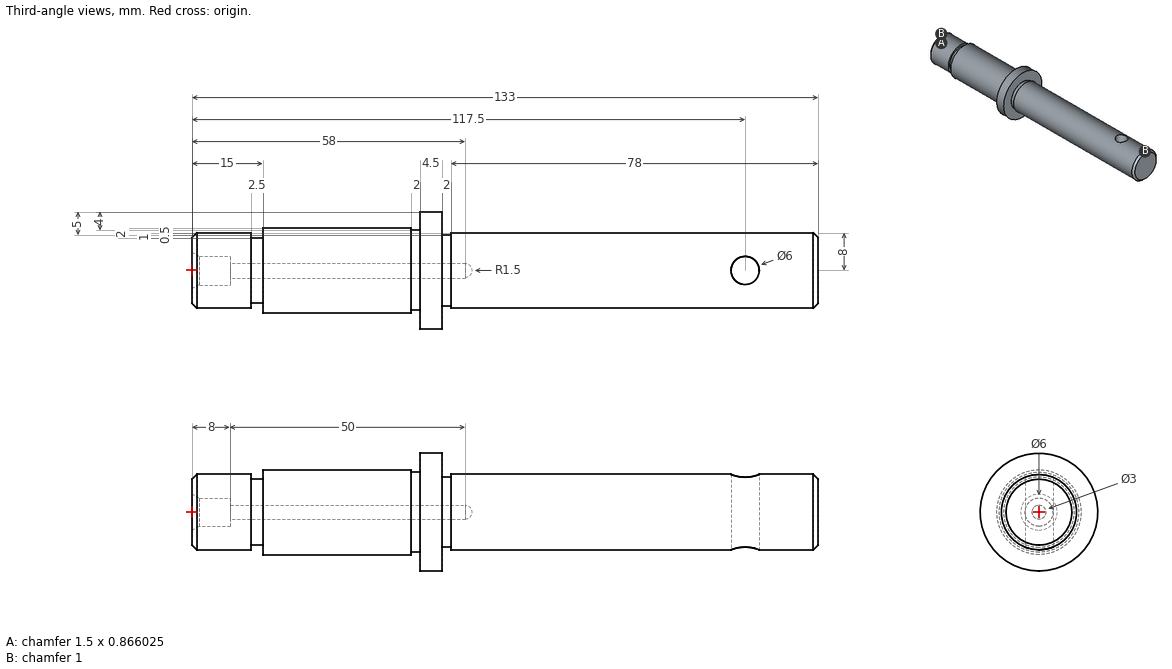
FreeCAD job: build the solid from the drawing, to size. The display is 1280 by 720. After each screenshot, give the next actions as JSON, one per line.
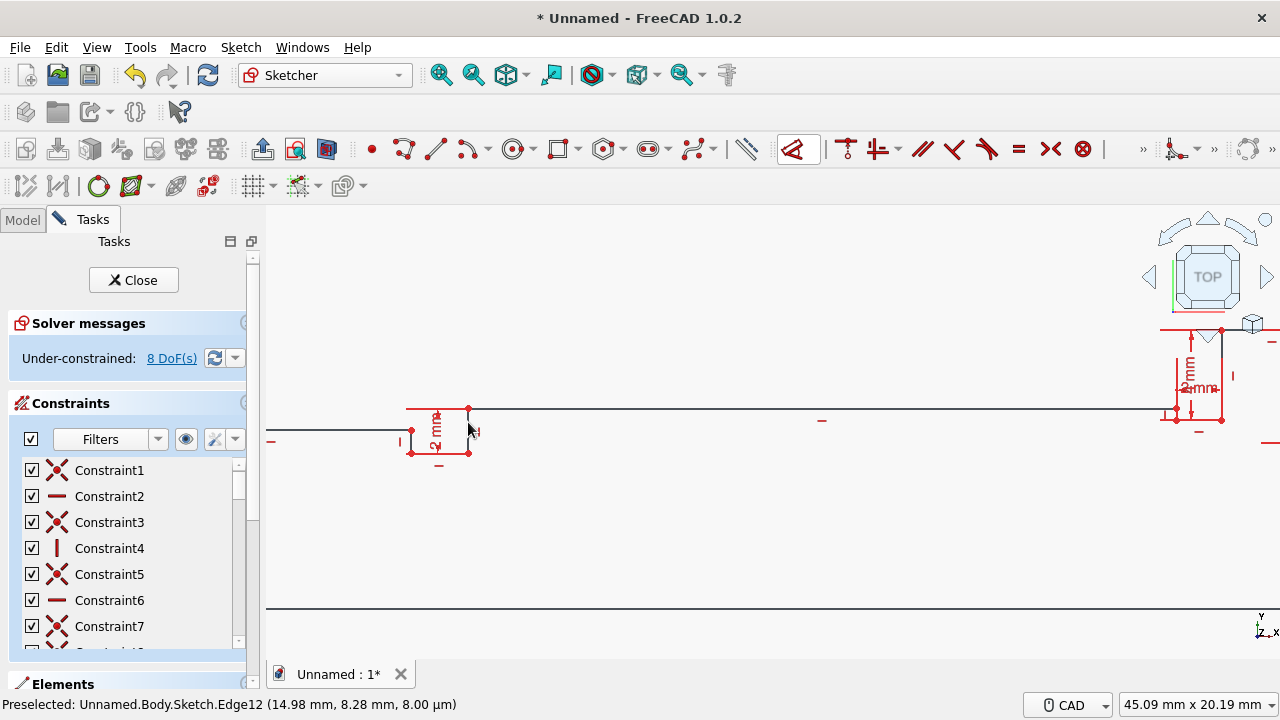
{"action": "scroll", "coordinate": [411, 444], "scroll_direction": "up", "scroll_amount": 3}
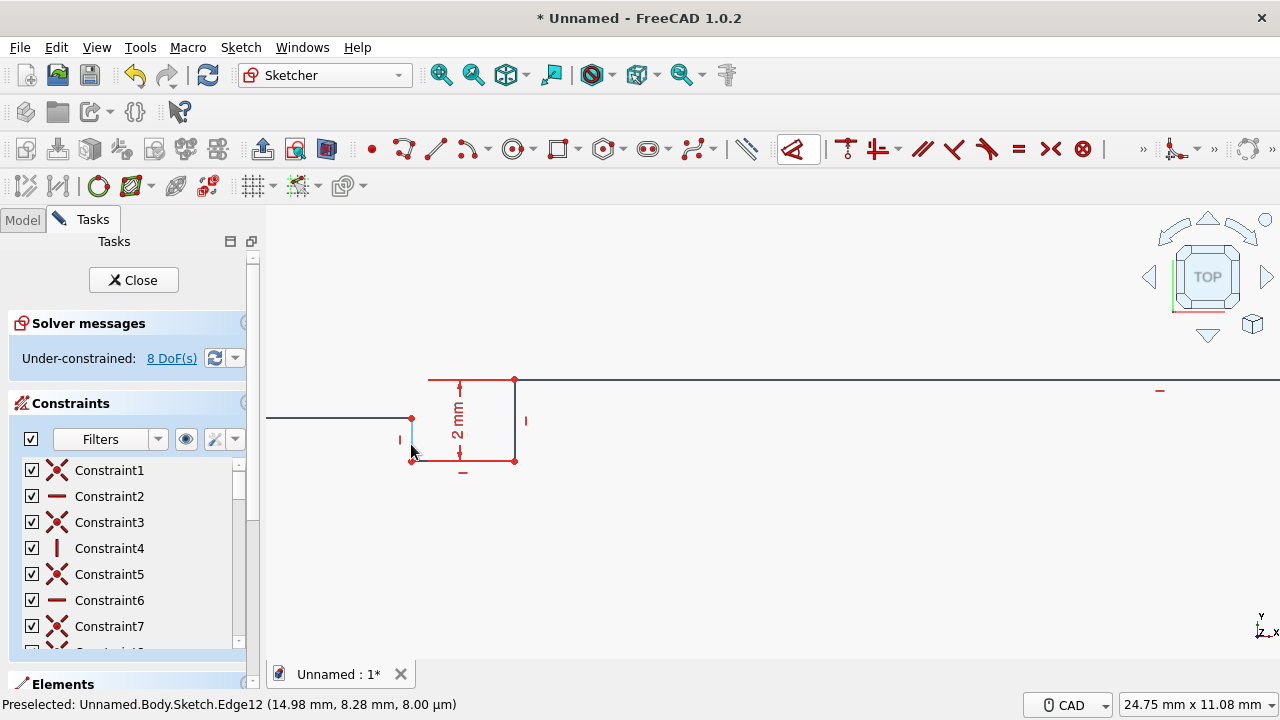
{"action": "left_click", "coordinate": [412, 444]}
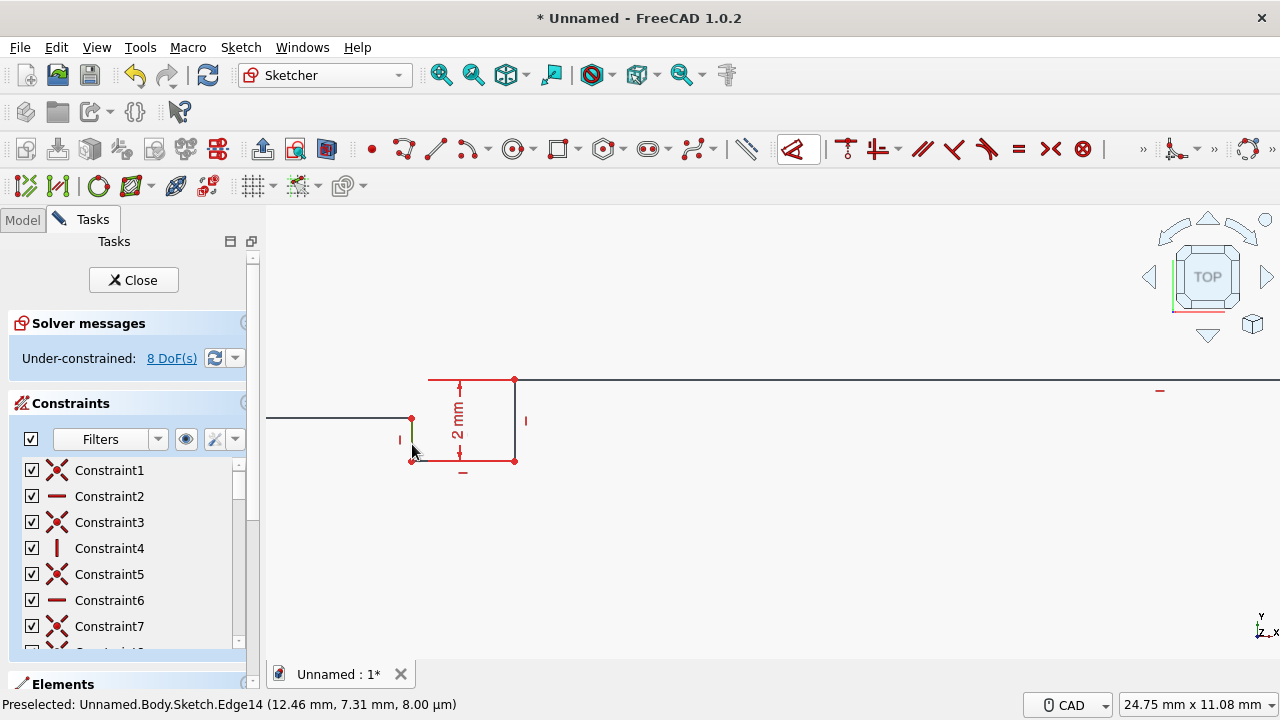
{"action": "key", "text": "i"}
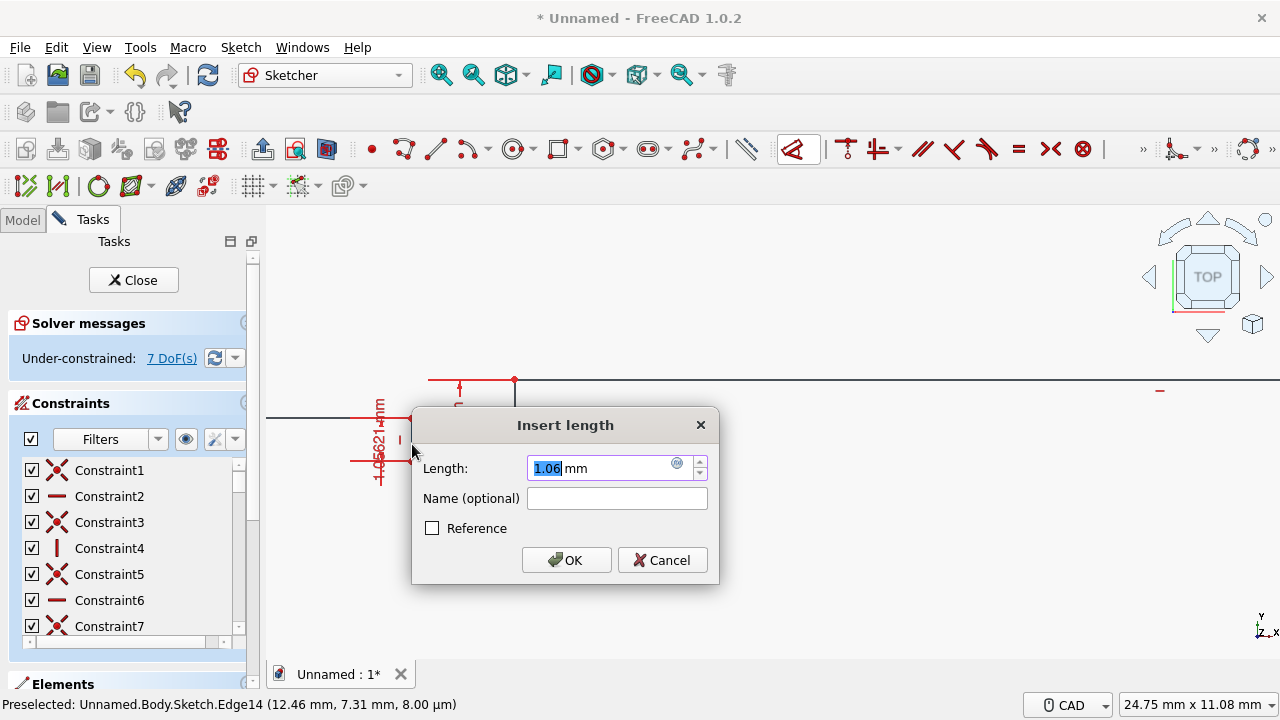
{"action": "type", "text": "1"}
{"action": "key", "text": "Return"}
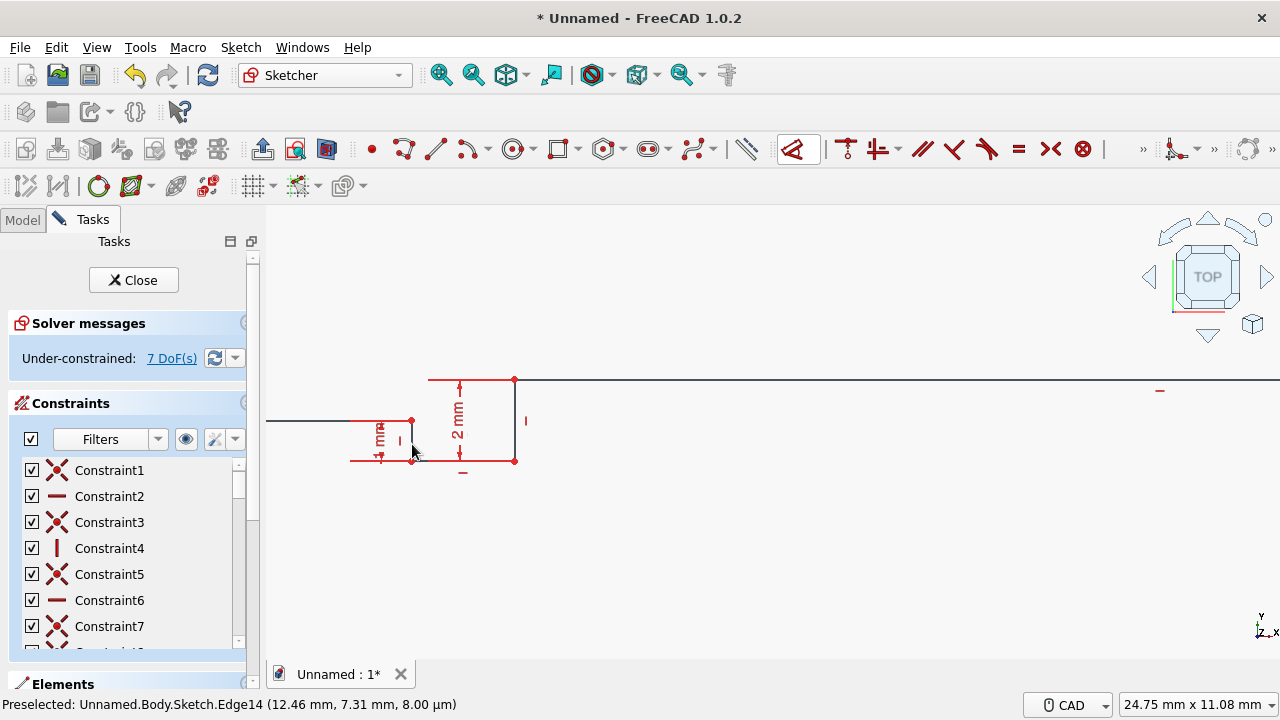
{"action": "scroll", "coordinate": [465, 425], "scroll_direction": "down", "scroll_amount": 11}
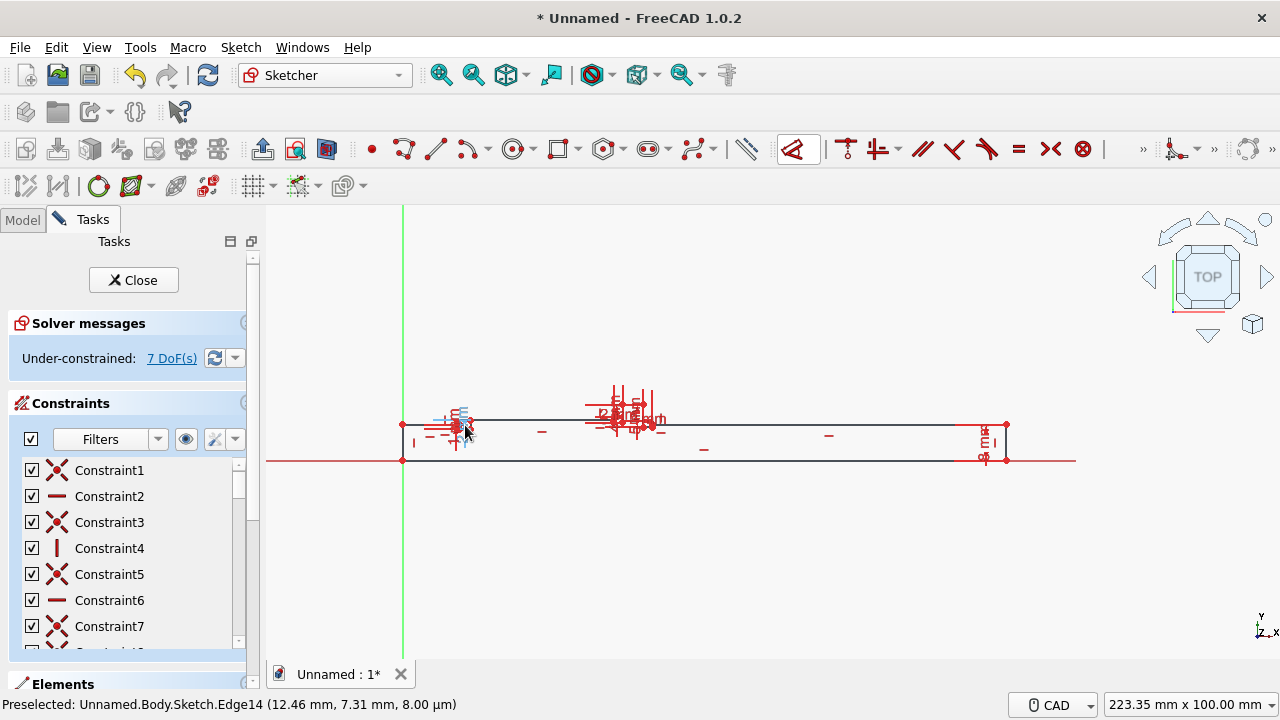
{"action": "scroll", "coordinate": [403, 436], "scroll_direction": "up", "scroll_amount": 2}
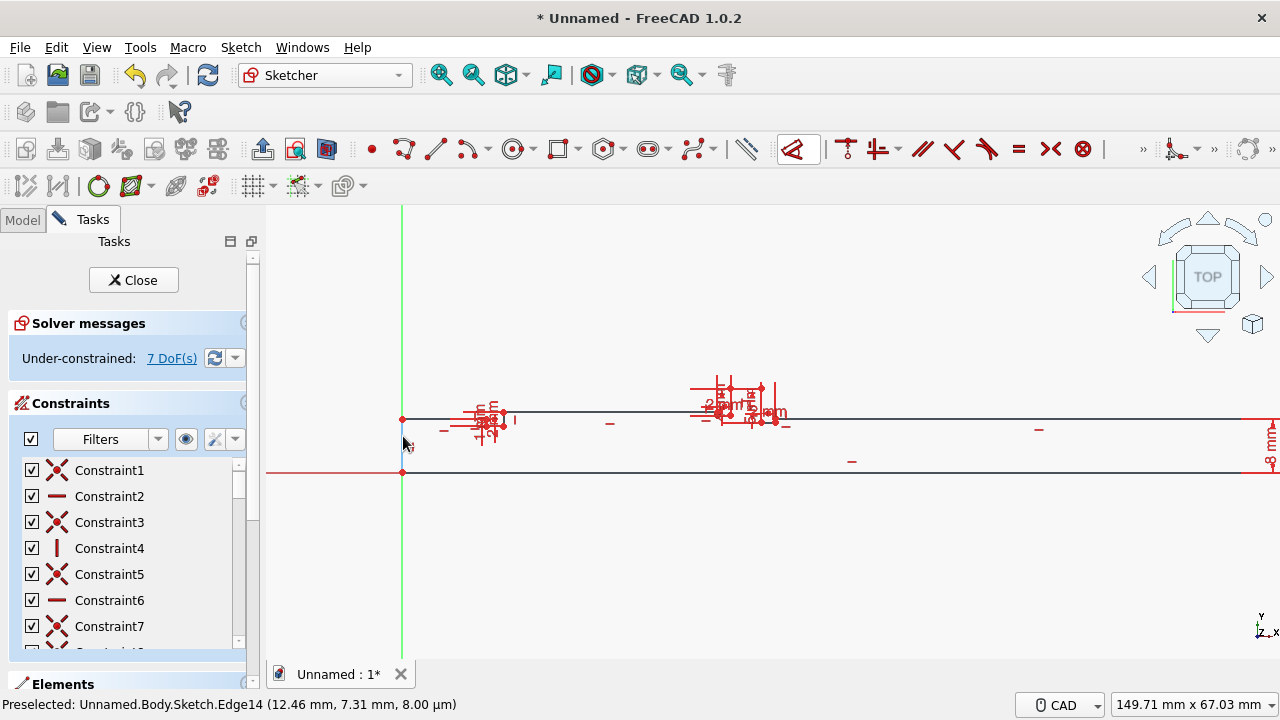
{"action": "left_click", "coordinate": [402, 435]}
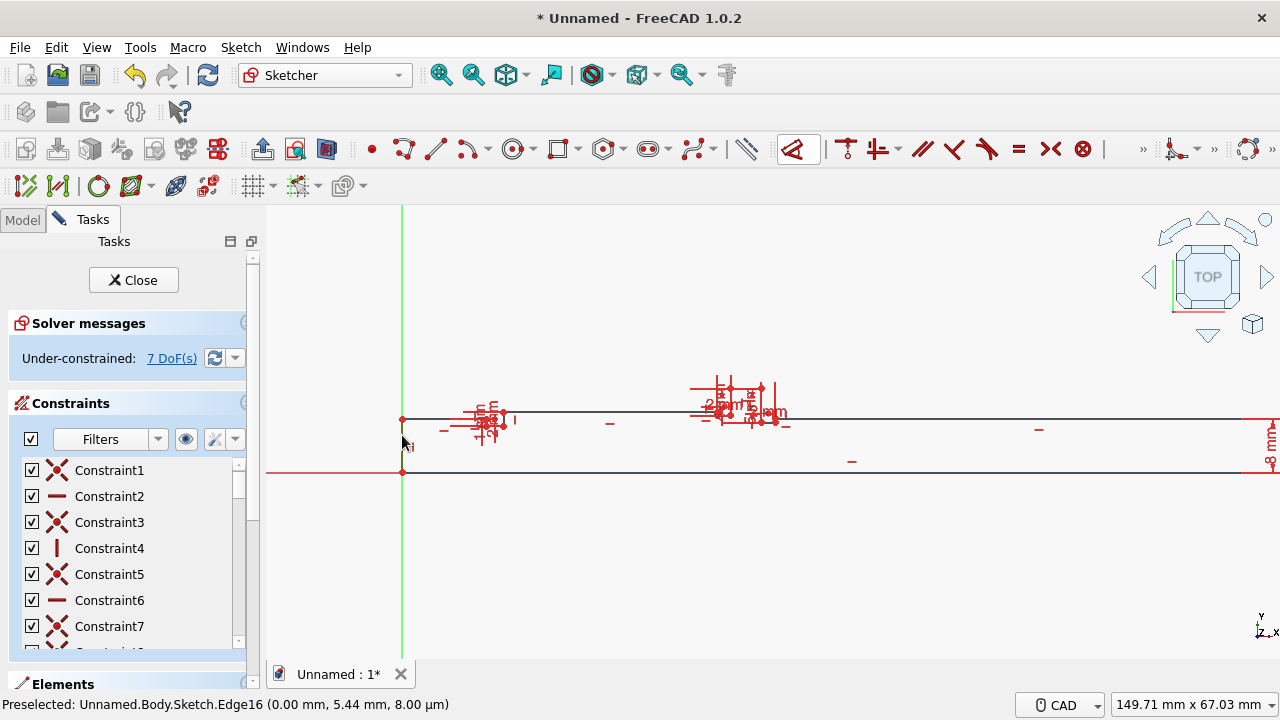
{"action": "left_click", "coordinate": [814, 150]}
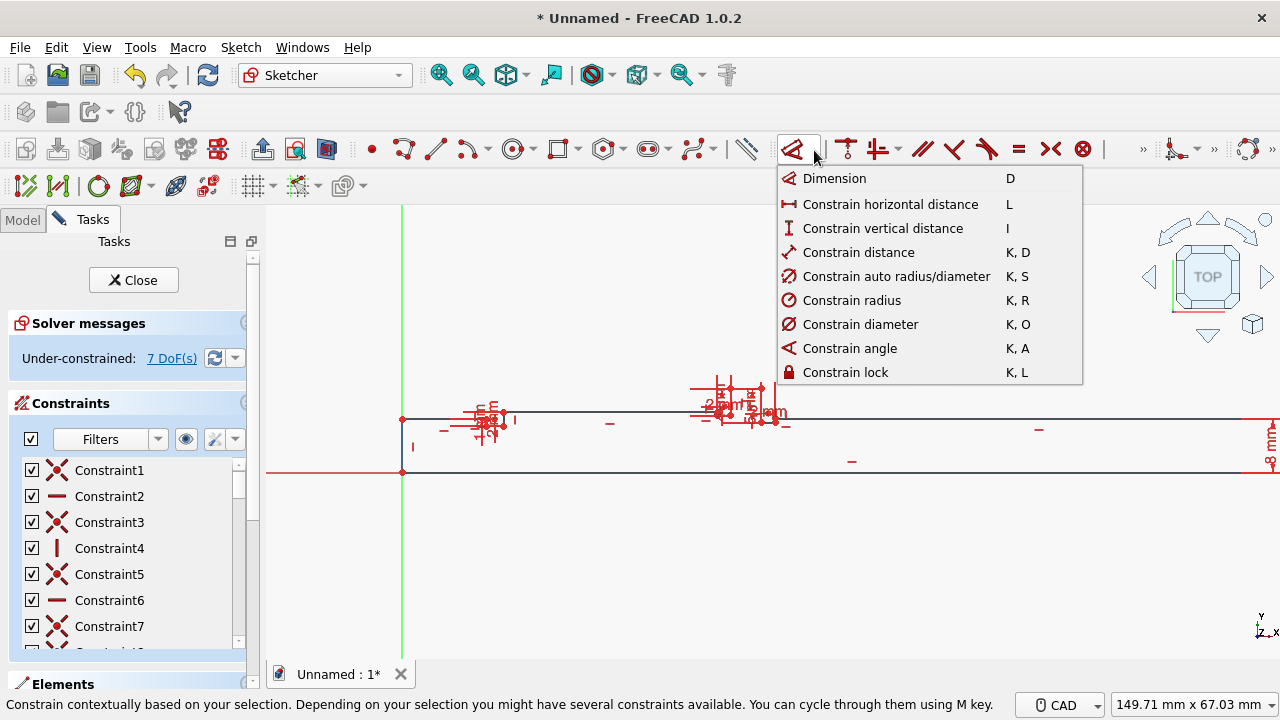
{"action": "left_click", "coordinate": [930, 228]}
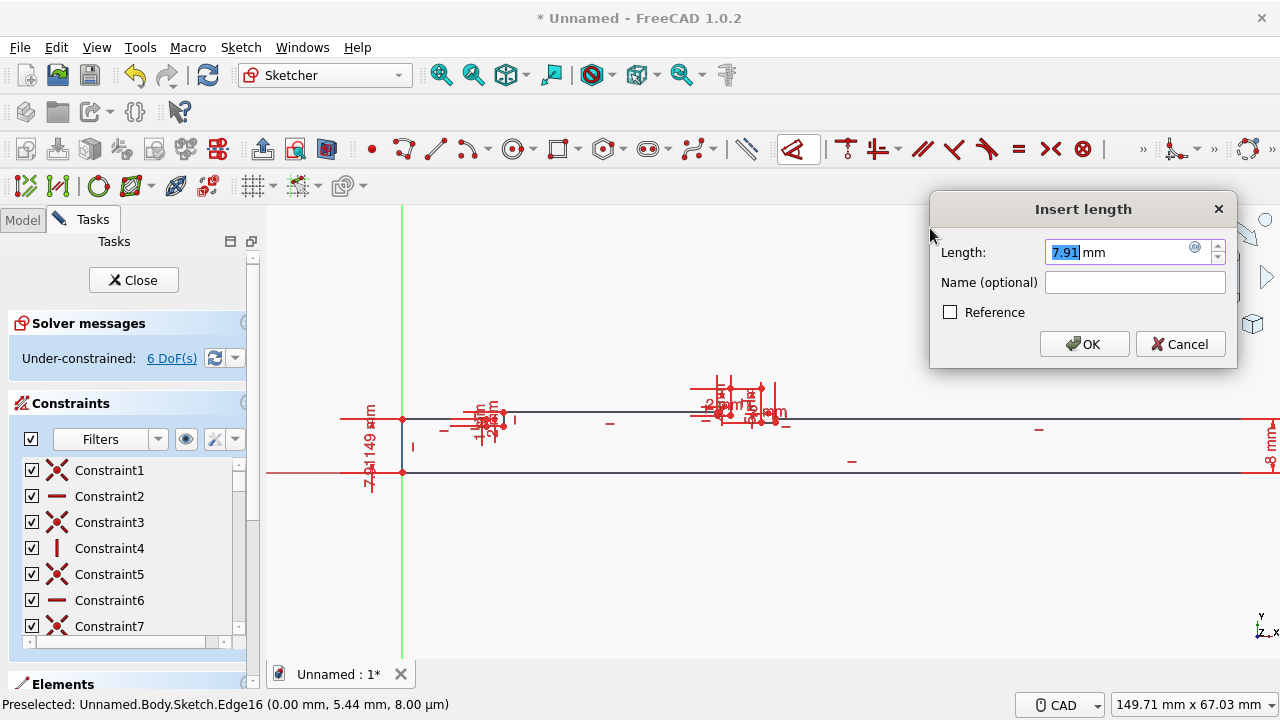
{"action": "type", "text": "8"}
{"action": "key", "text": "Return"}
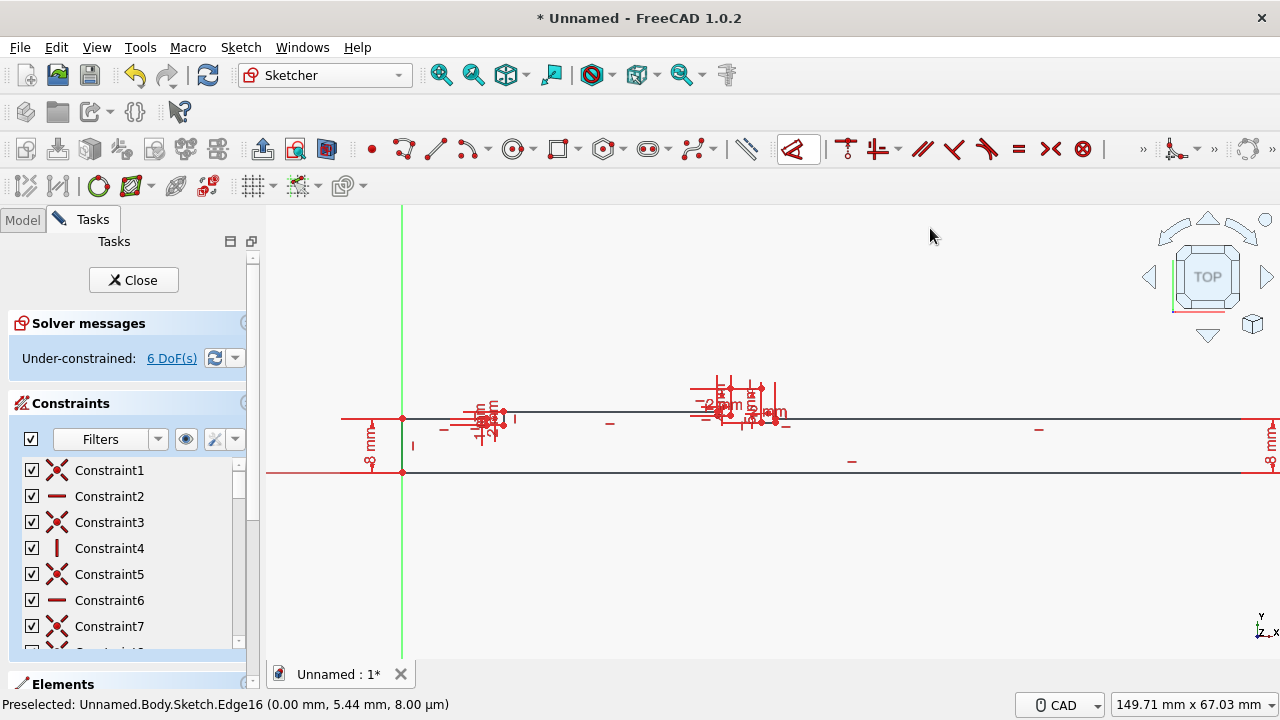
{"action": "left_click", "coordinate": [933, 419]}